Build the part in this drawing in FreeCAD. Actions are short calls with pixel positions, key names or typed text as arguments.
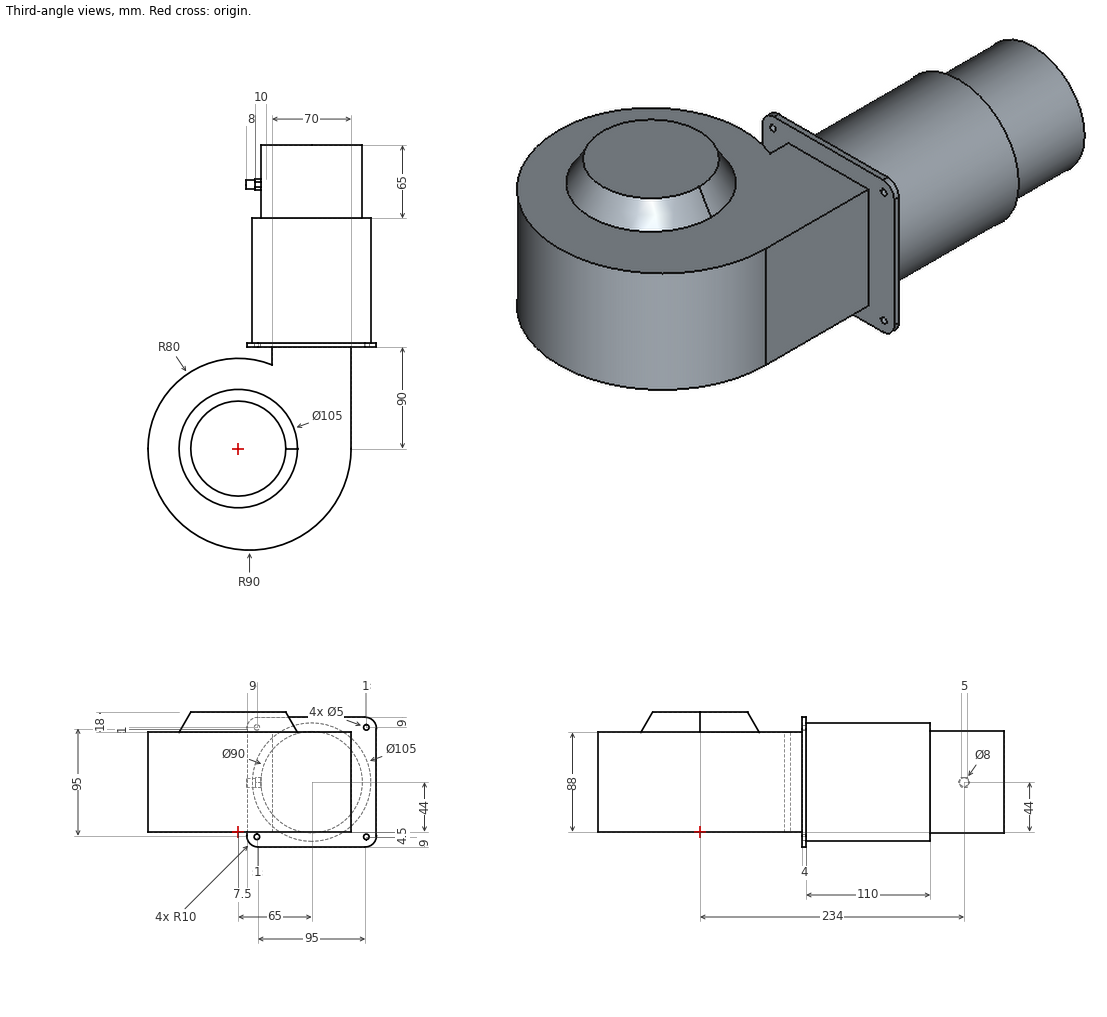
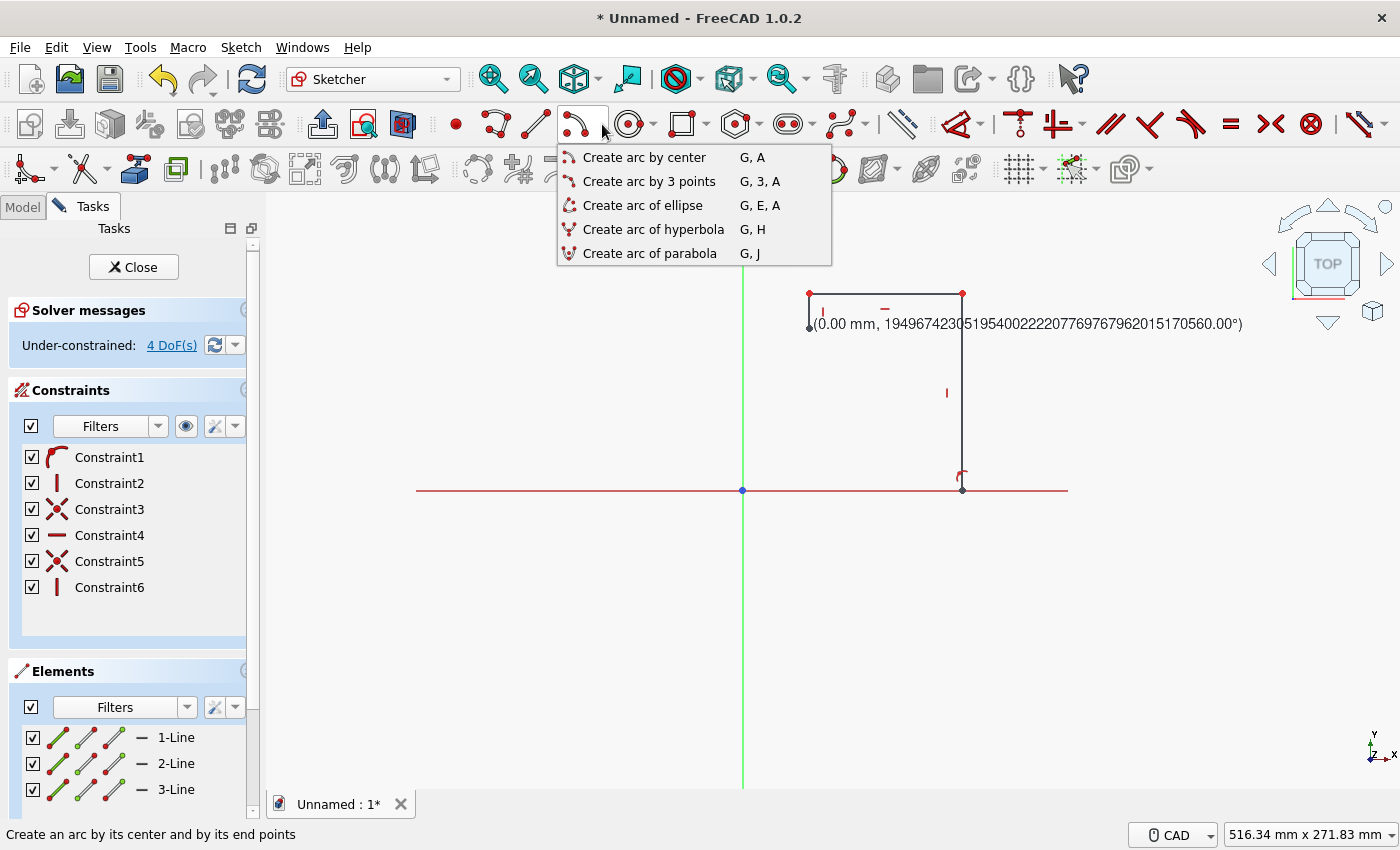
click(694, 181)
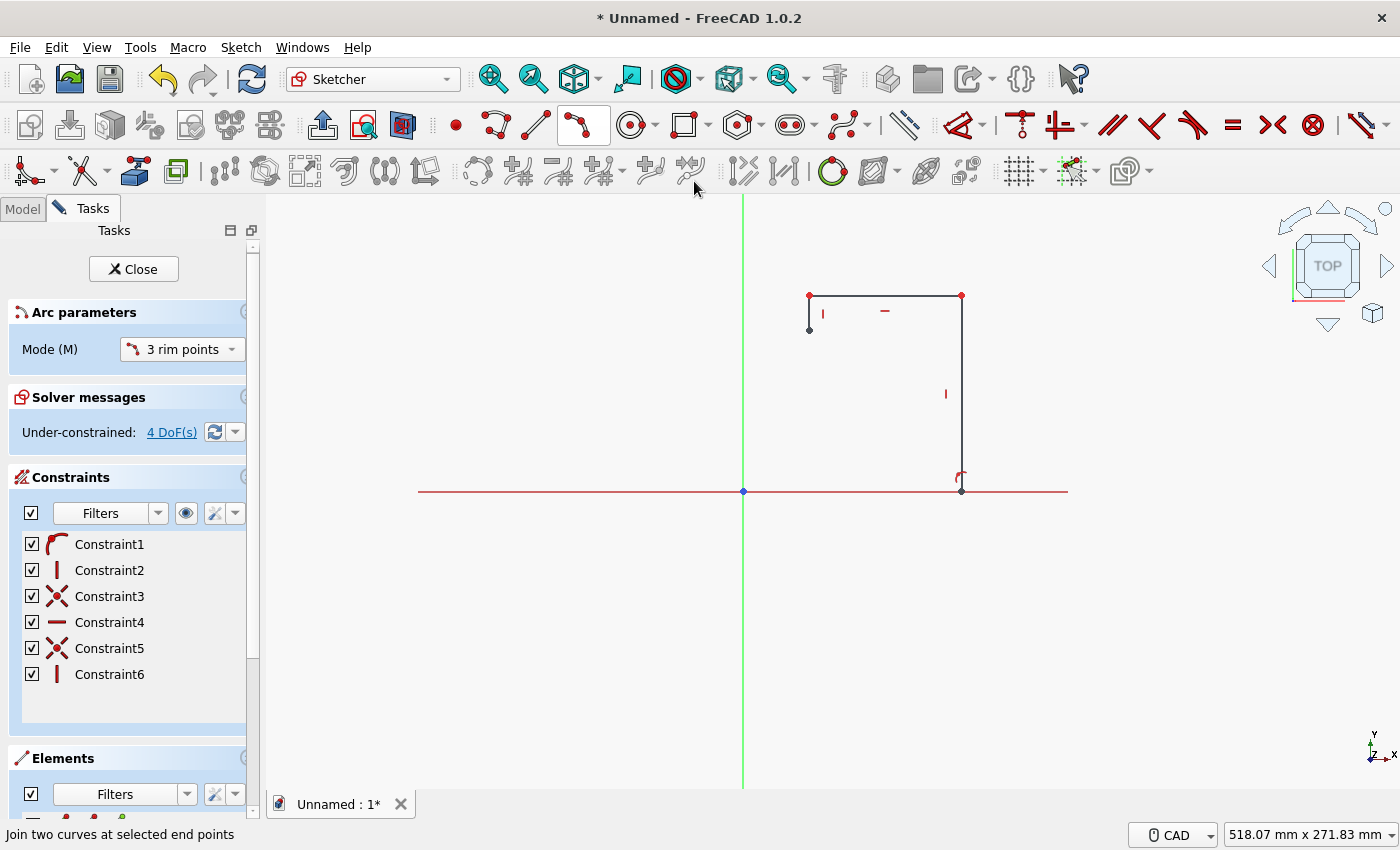
click(809, 331)
click(568, 492)
click(645, 346)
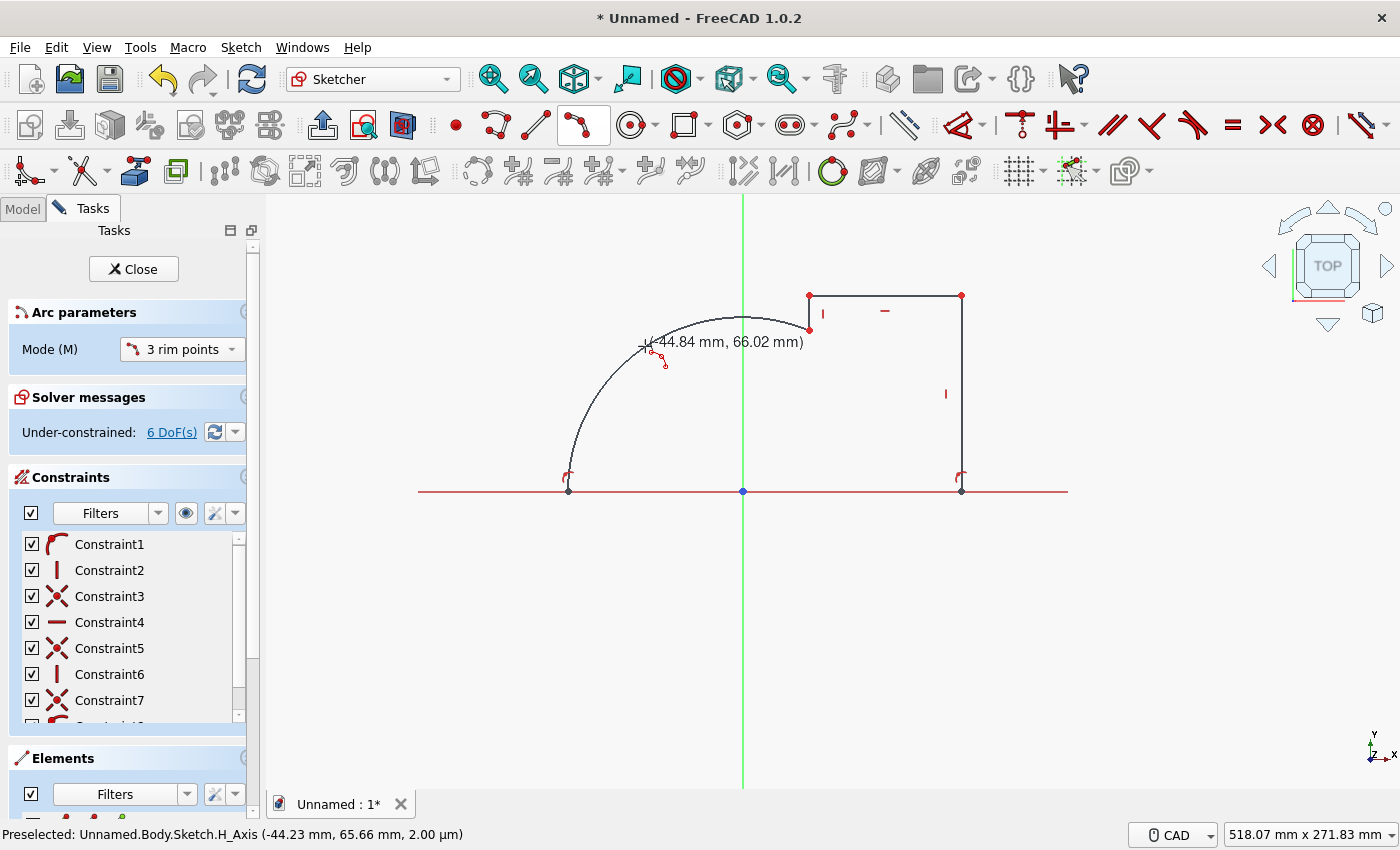
click(568, 492)
click(962, 492)
click(765, 688)
key(Escape)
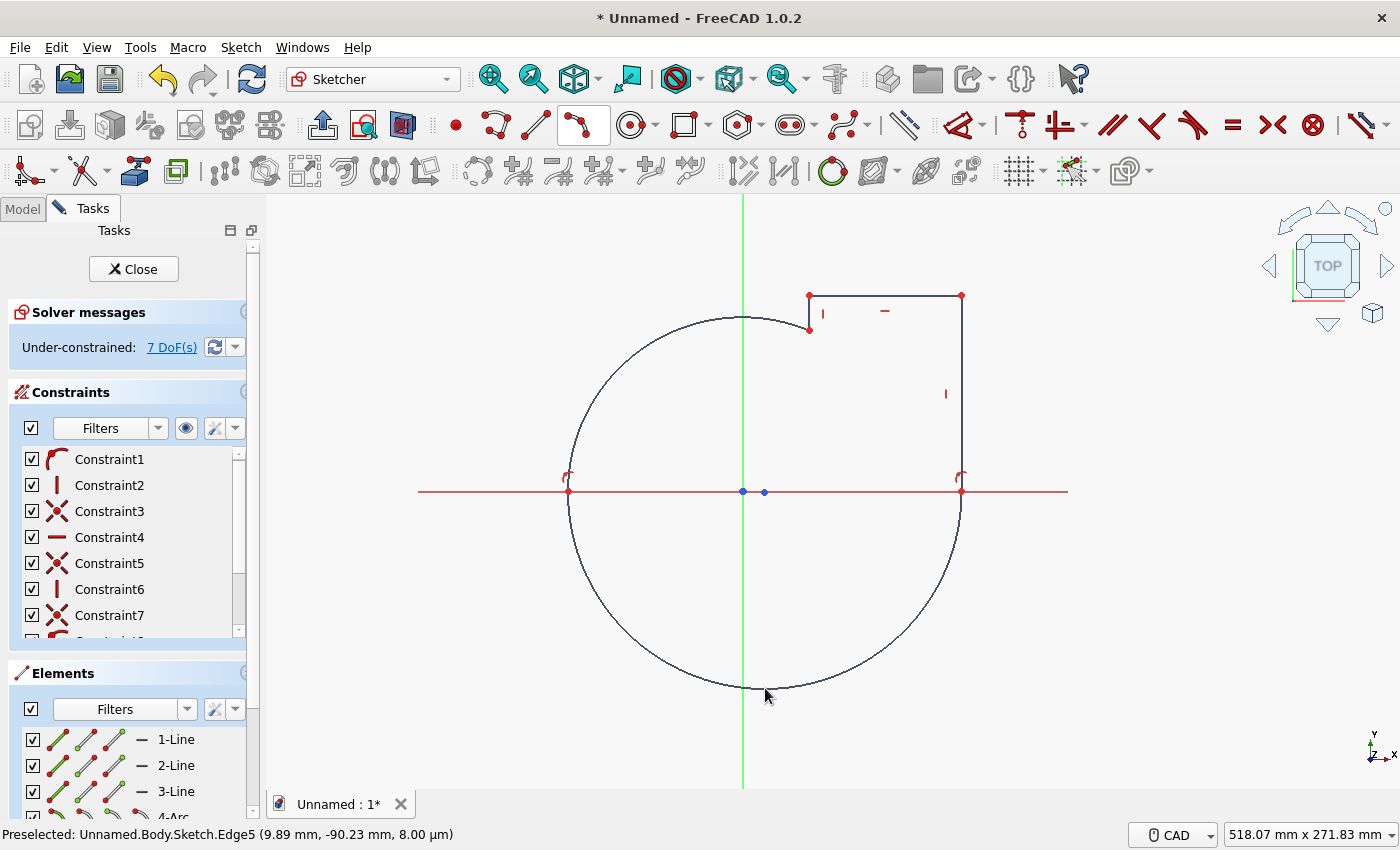
drag(732, 482, 753, 502)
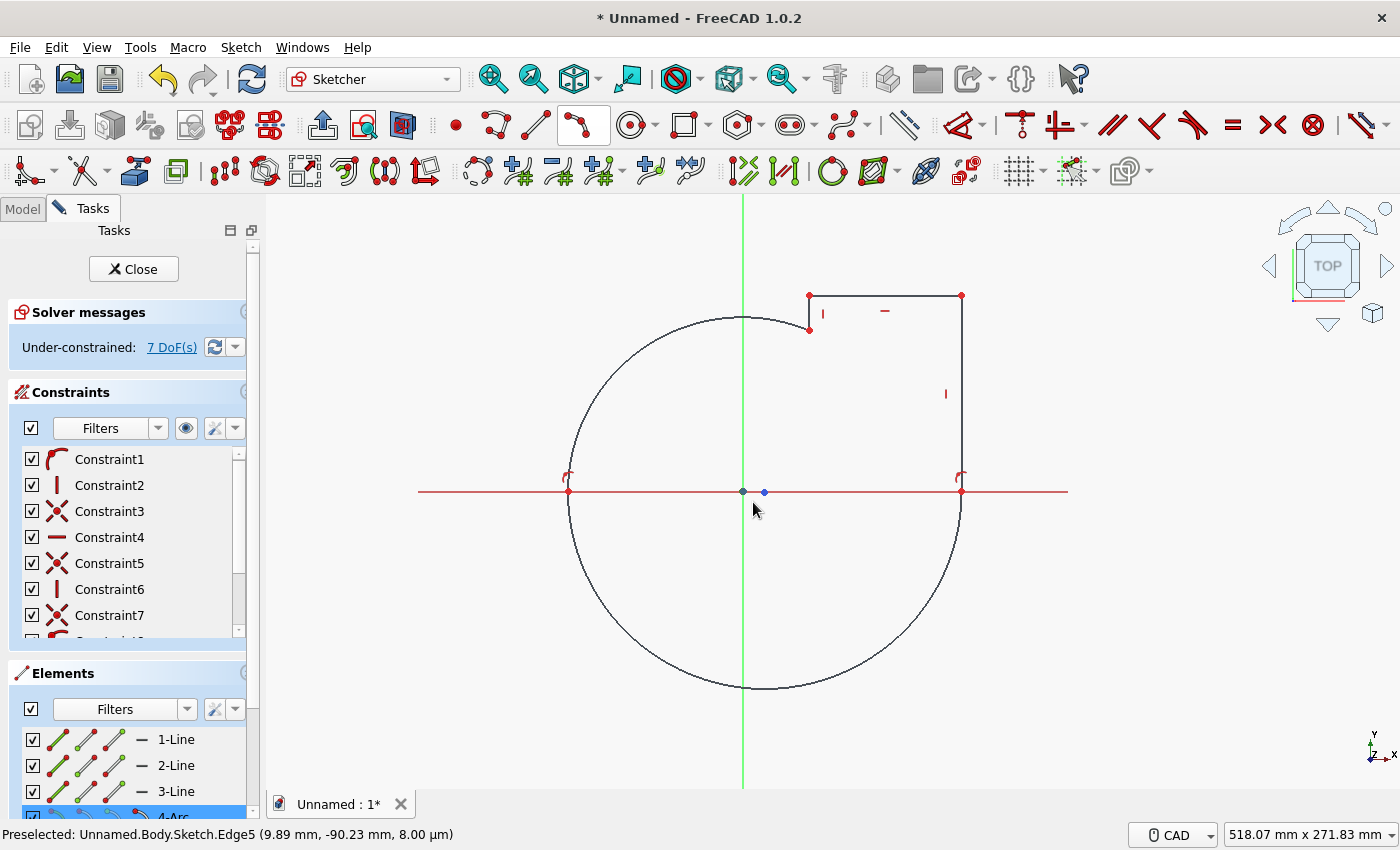
click(1020, 126)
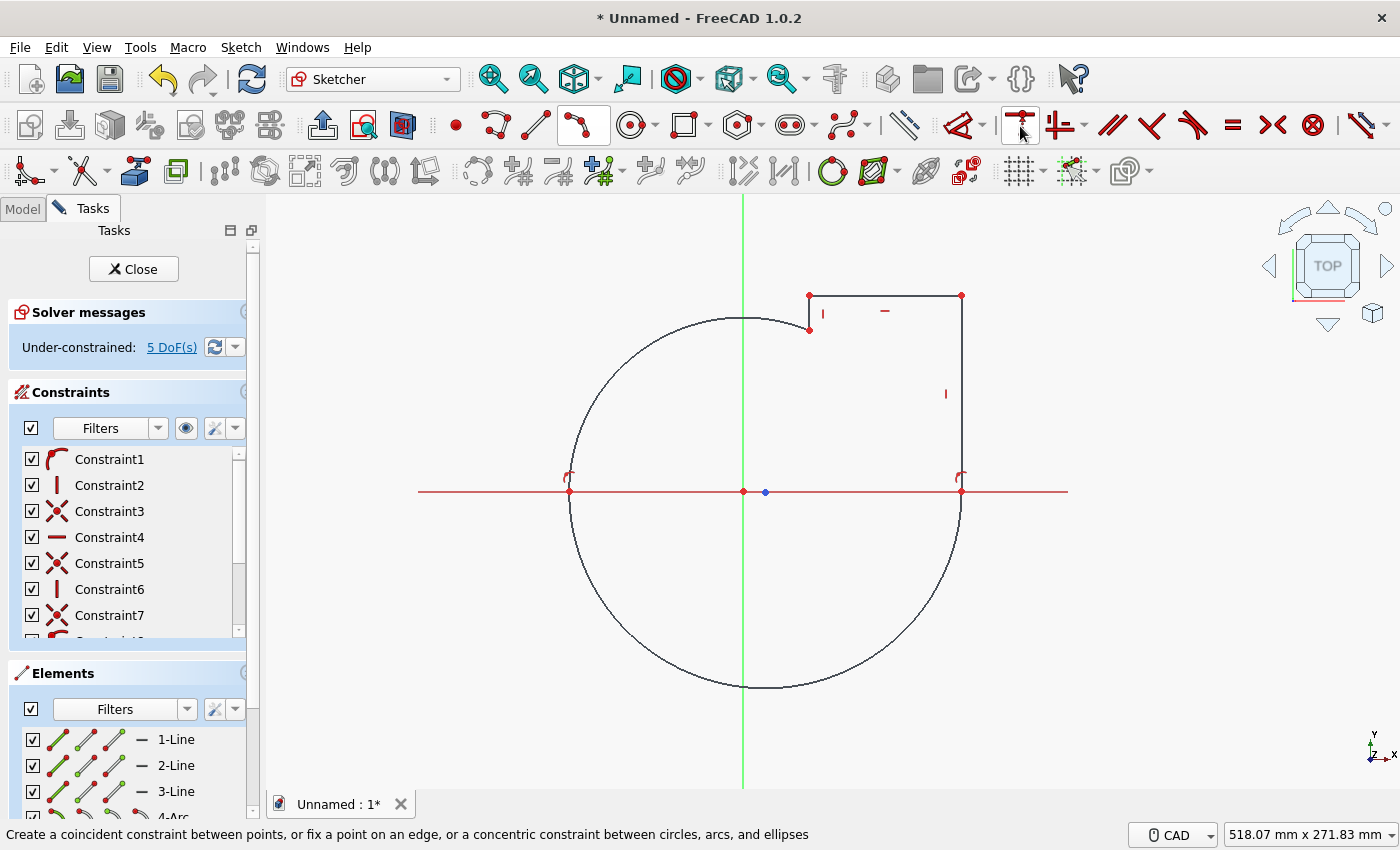
click(765, 492)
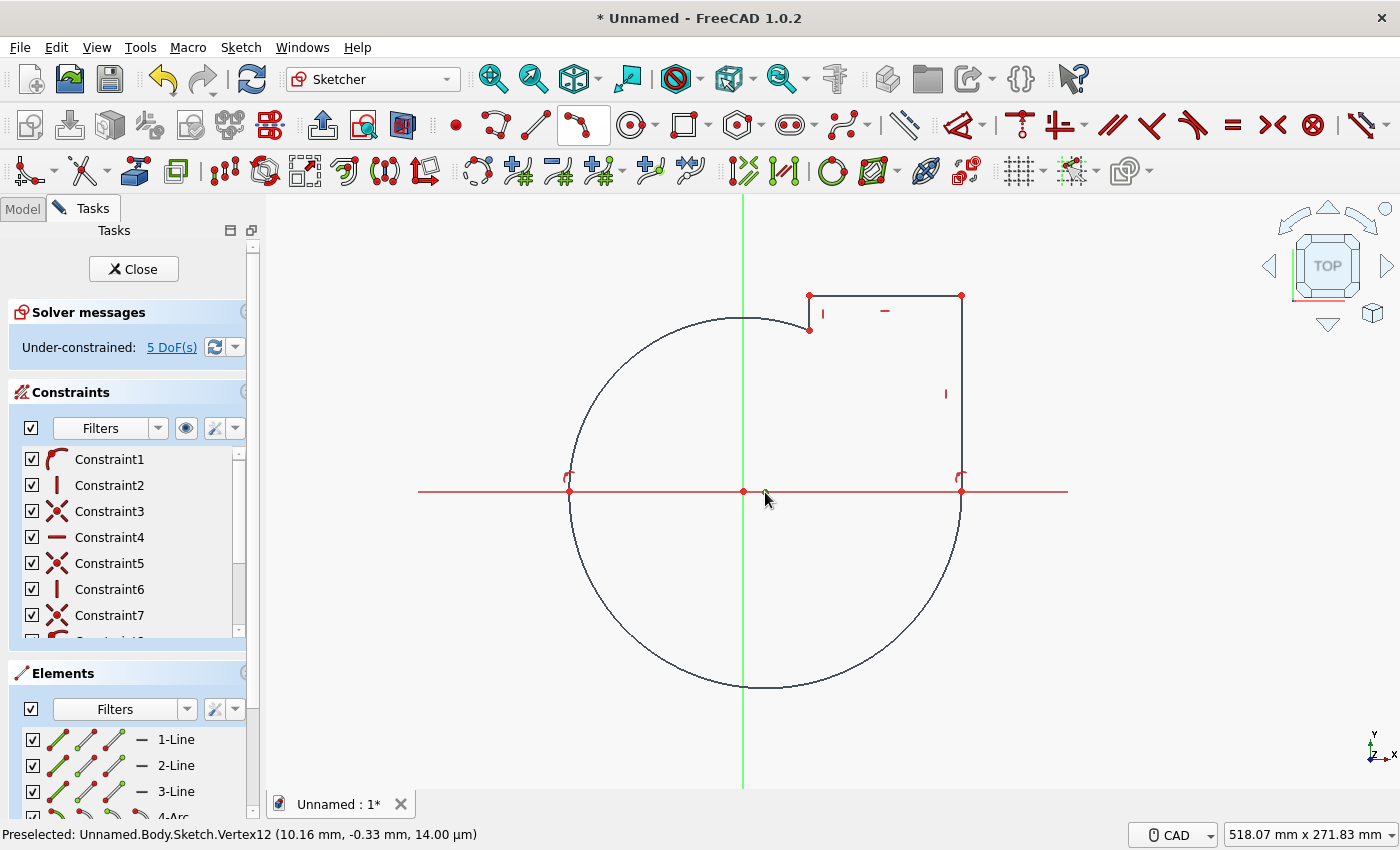
click(428, 492)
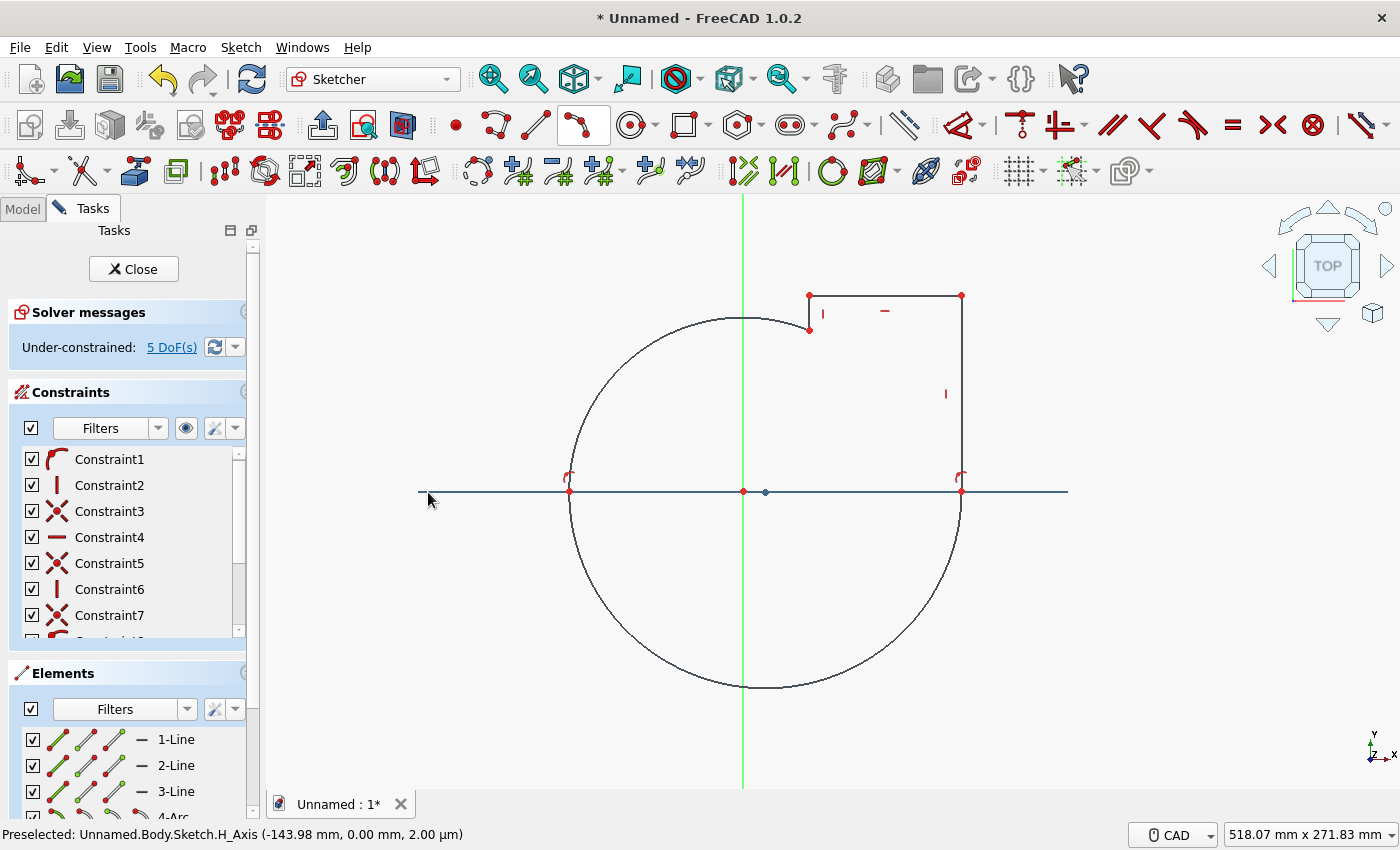
key(c)